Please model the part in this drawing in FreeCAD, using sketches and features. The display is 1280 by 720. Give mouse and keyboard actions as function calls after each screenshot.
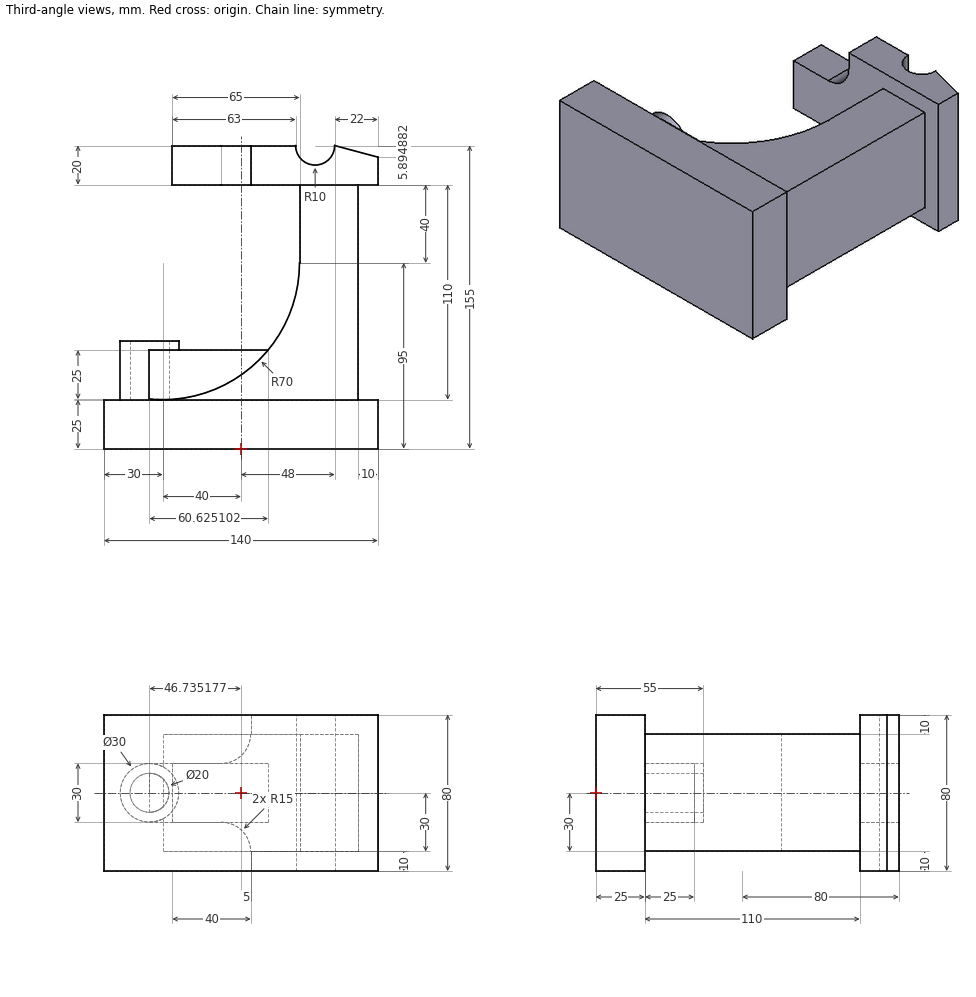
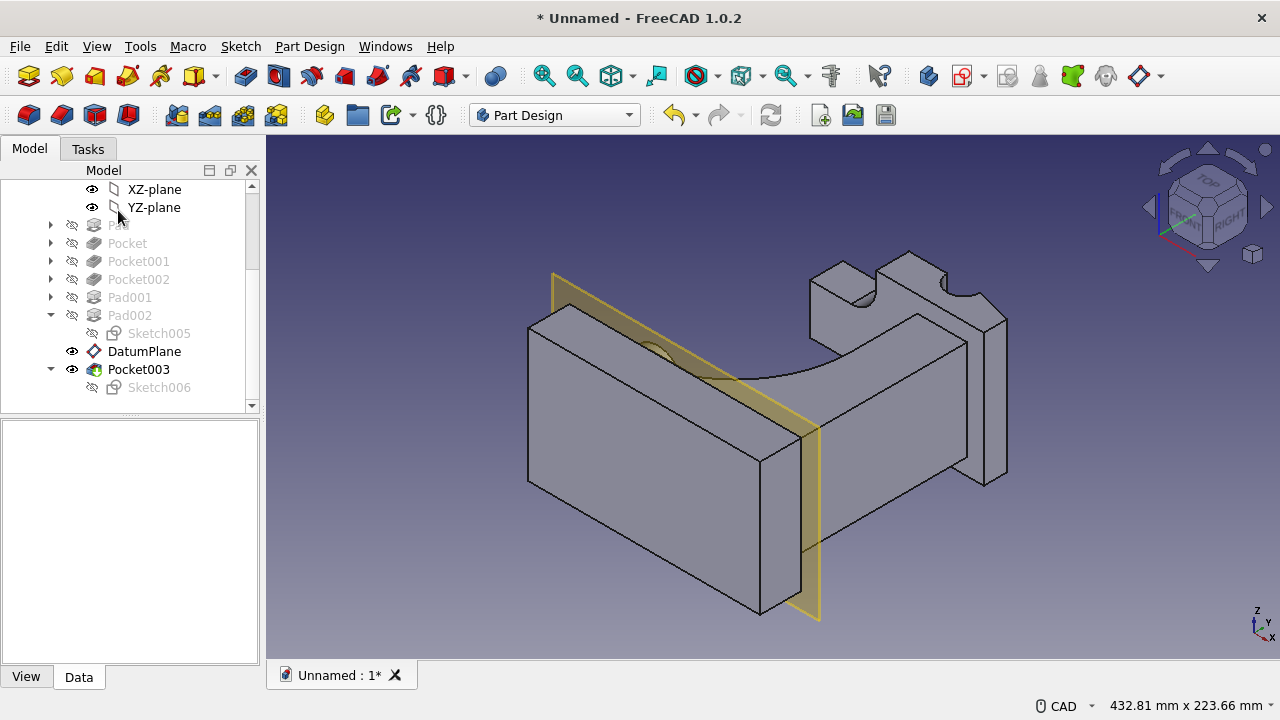
click(117, 351)
key(space)